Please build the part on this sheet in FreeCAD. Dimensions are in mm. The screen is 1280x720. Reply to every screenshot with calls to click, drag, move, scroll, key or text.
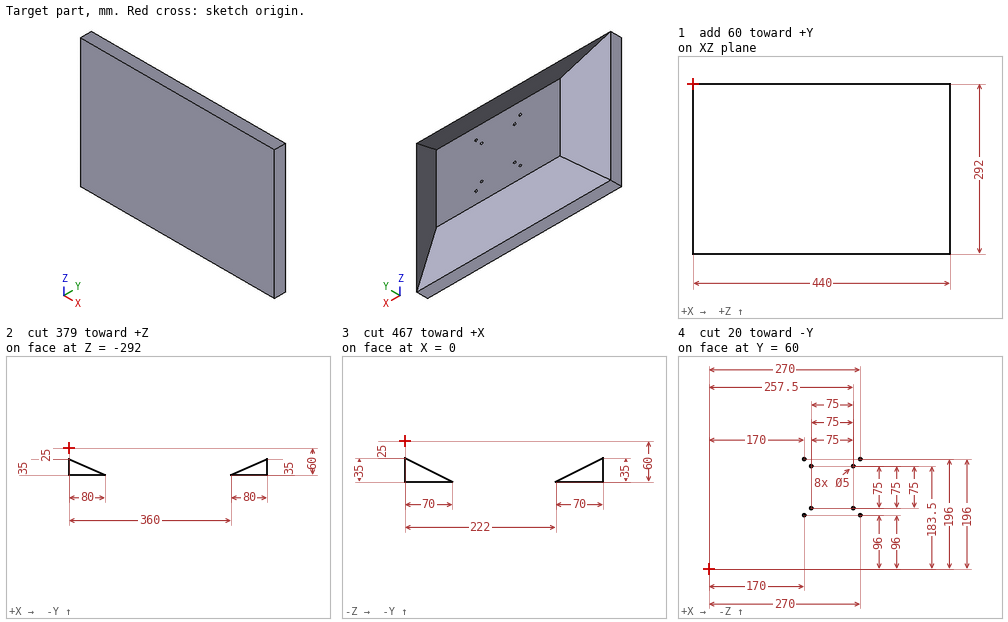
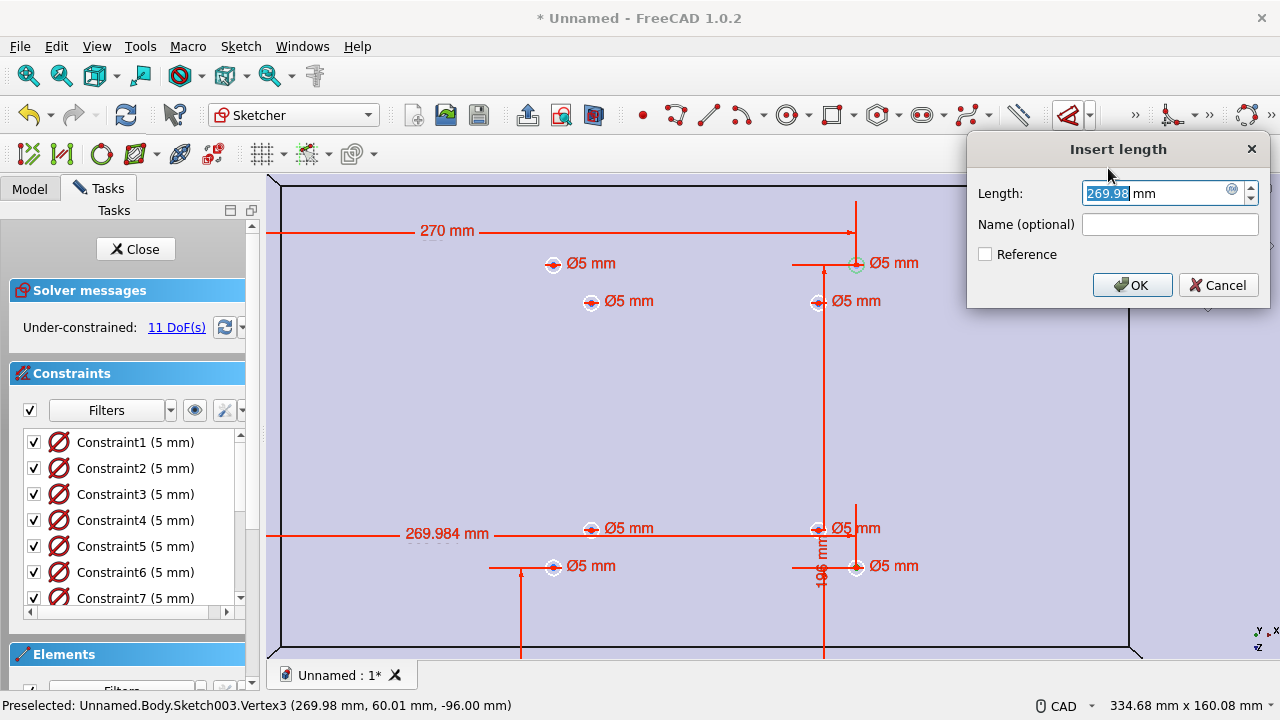
text(270)
key(Return)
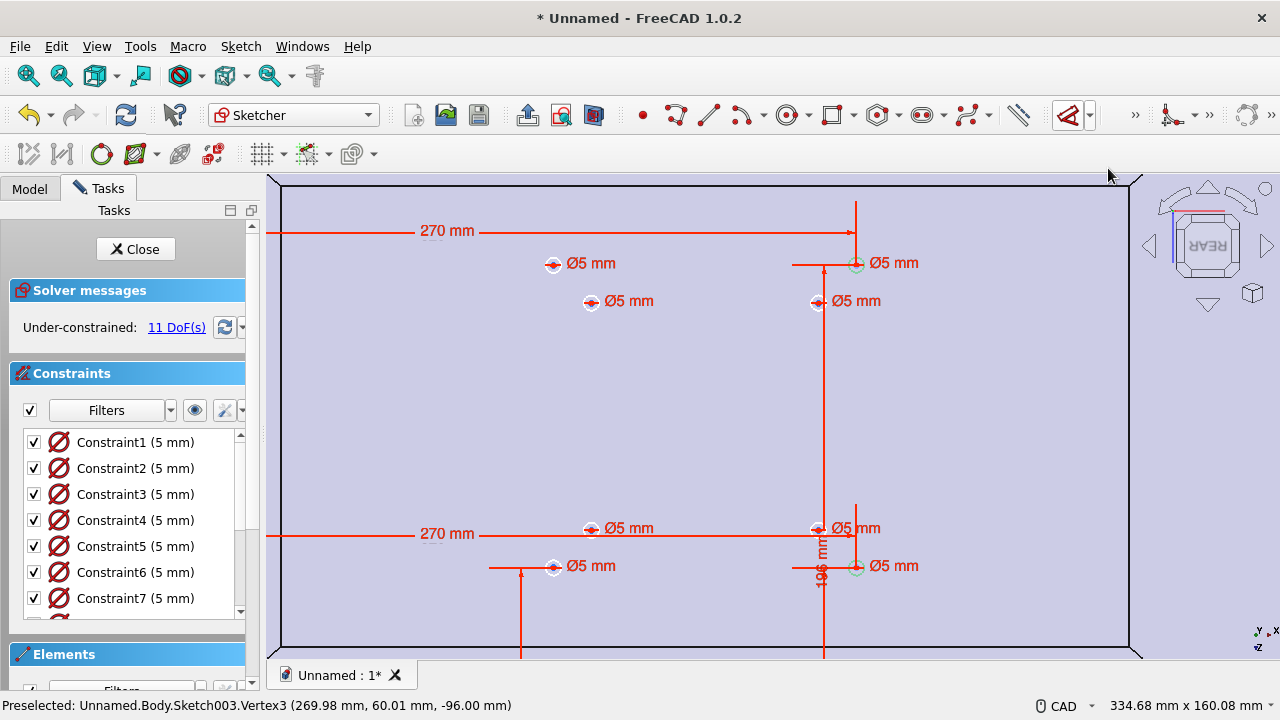
click(553, 568)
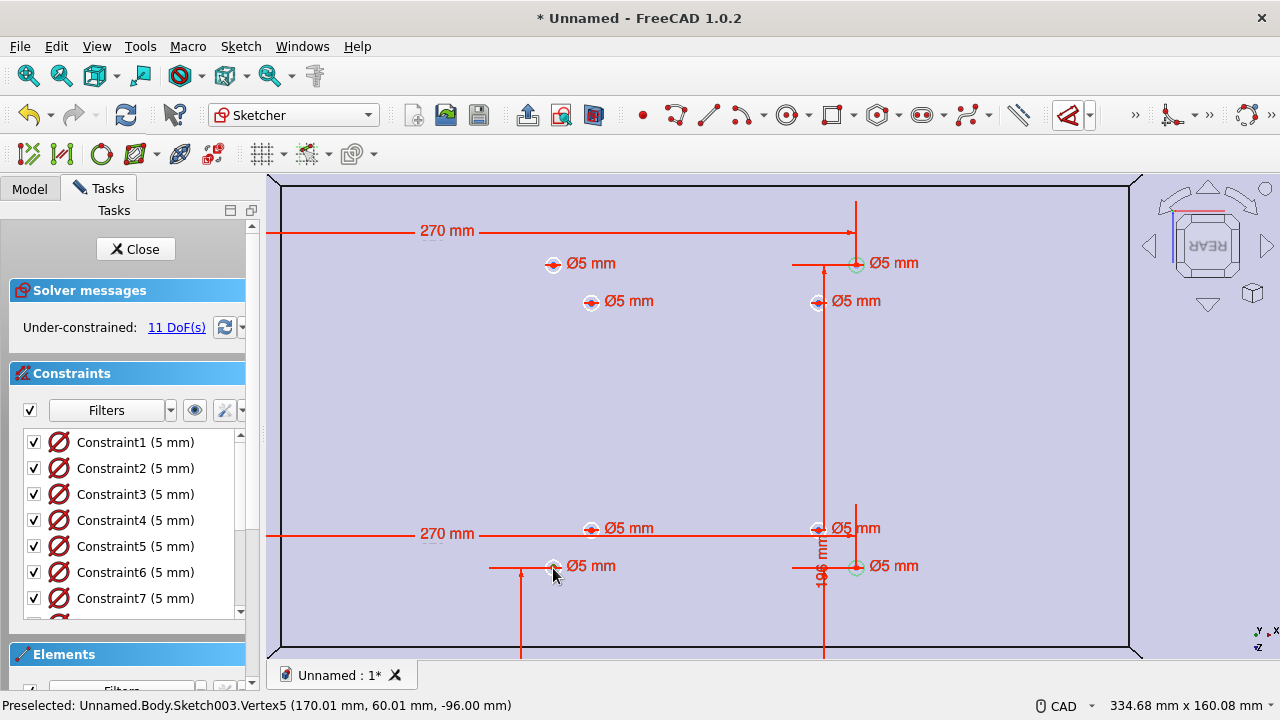
key(l)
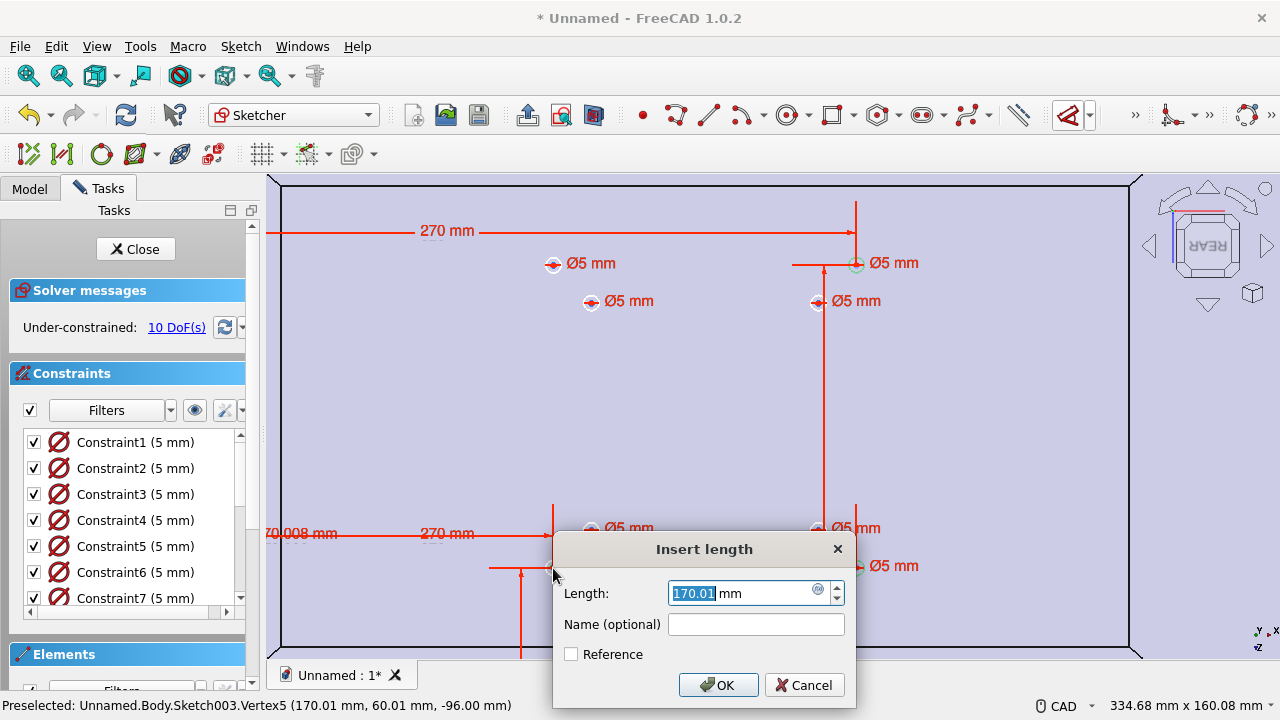
text(170)
key(Return)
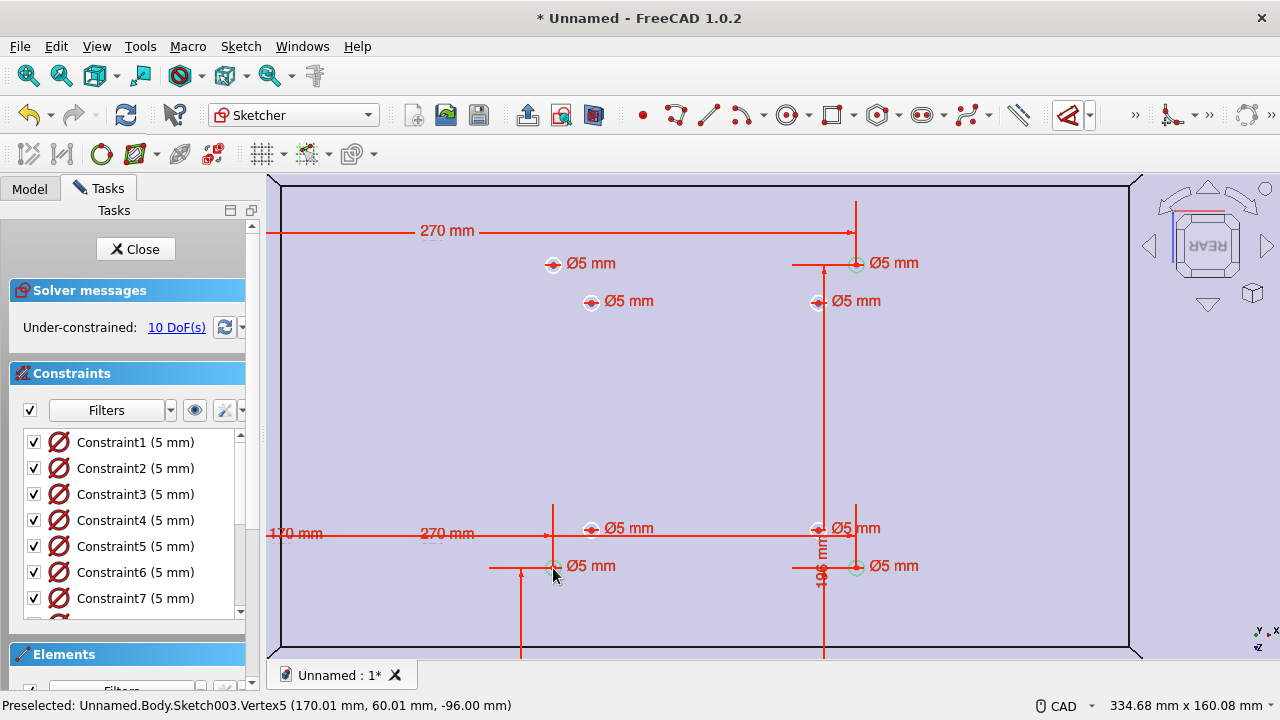
click(553, 265)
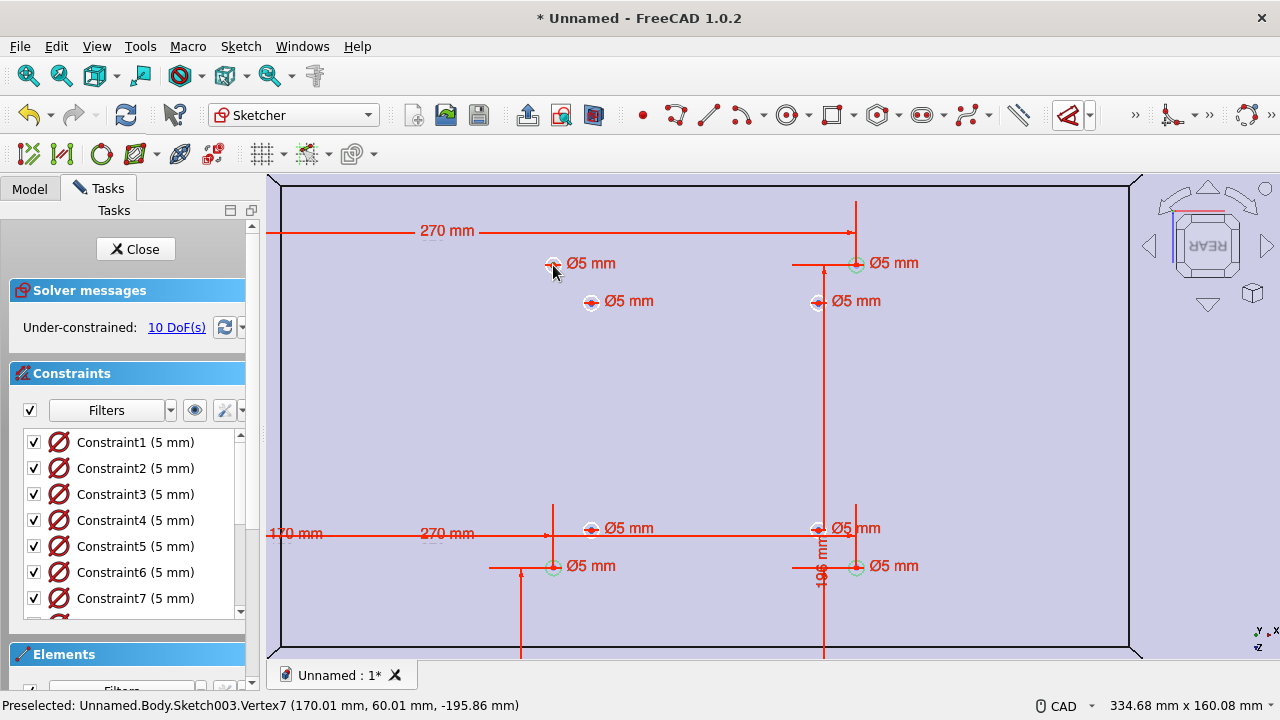
key(l)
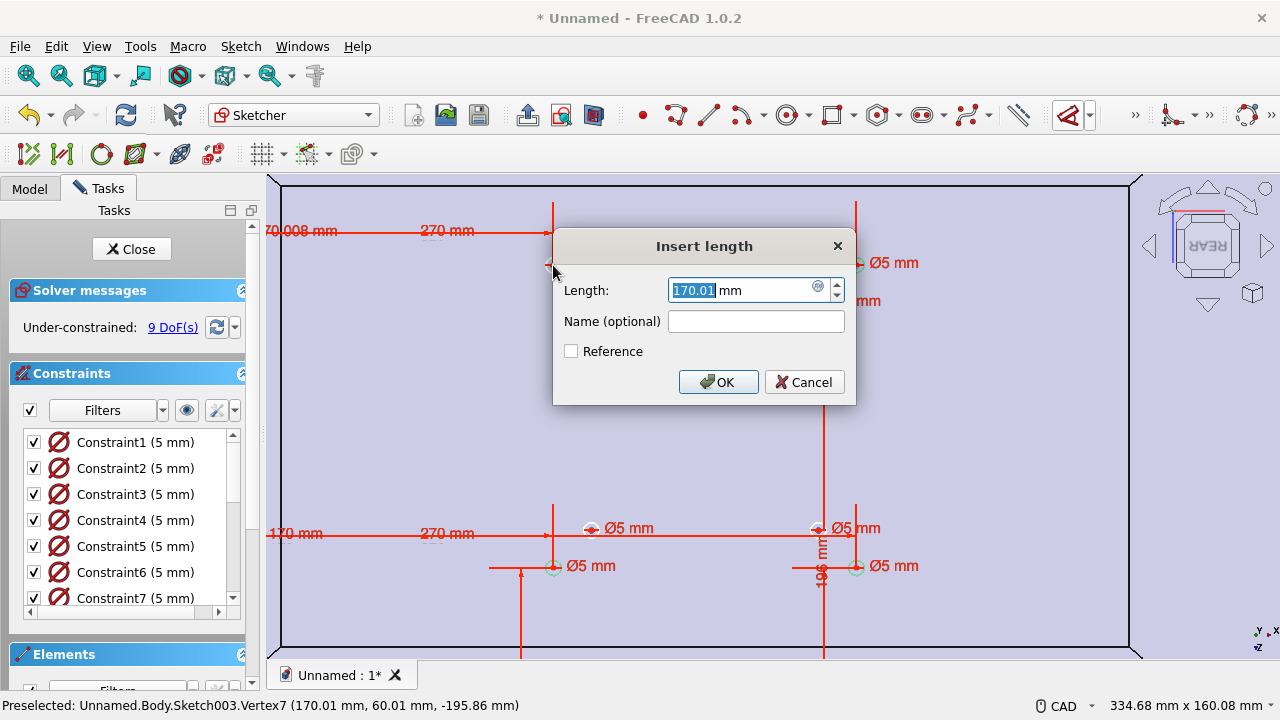
text(170)
key(Return)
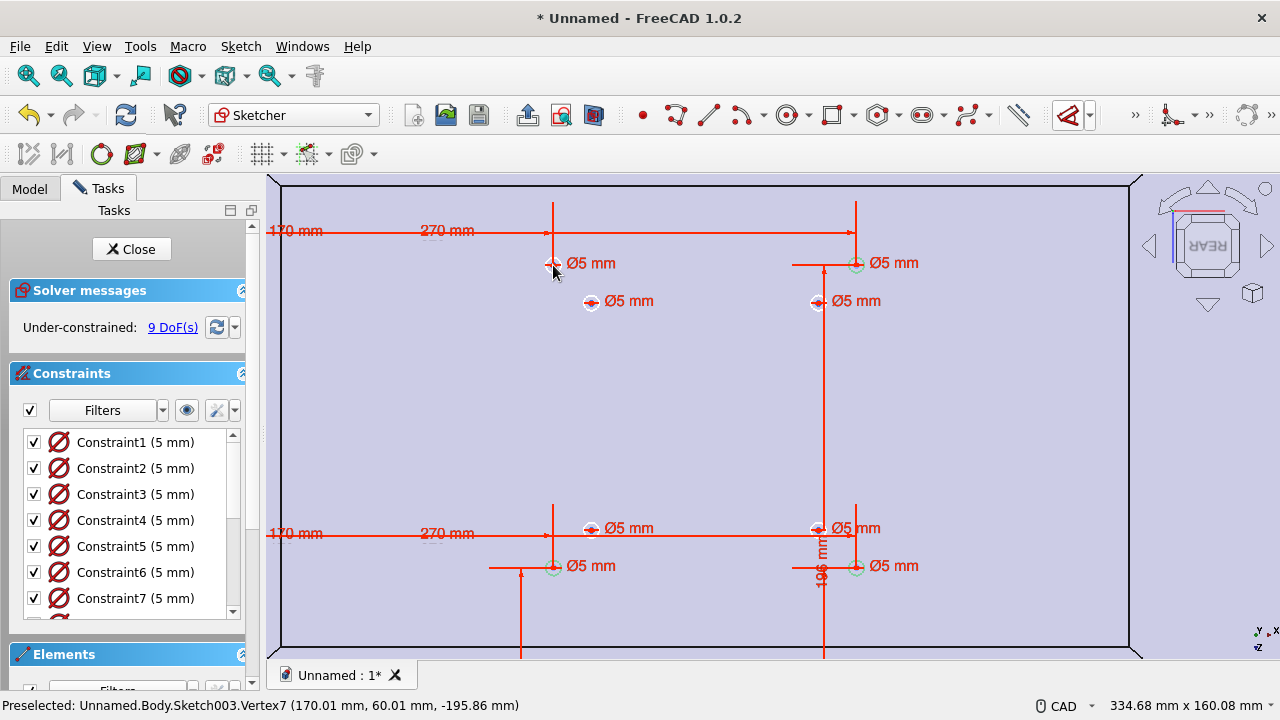
click(553, 265)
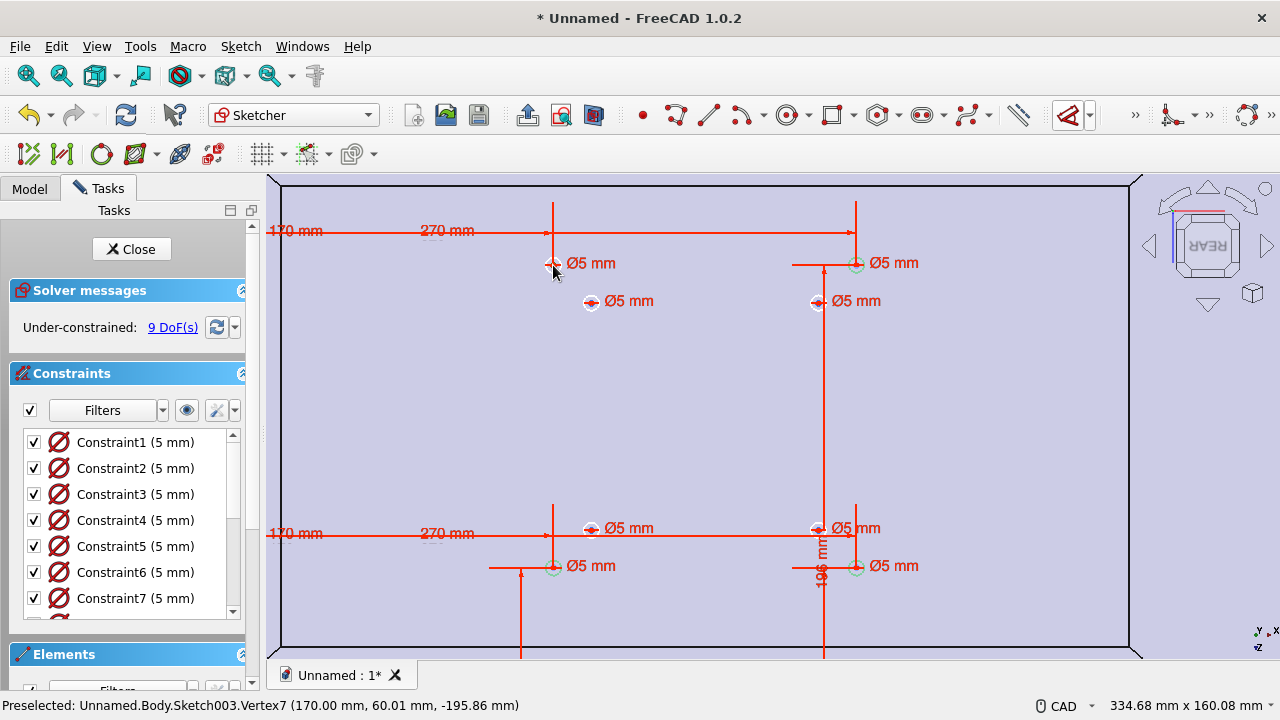
click(1090, 116)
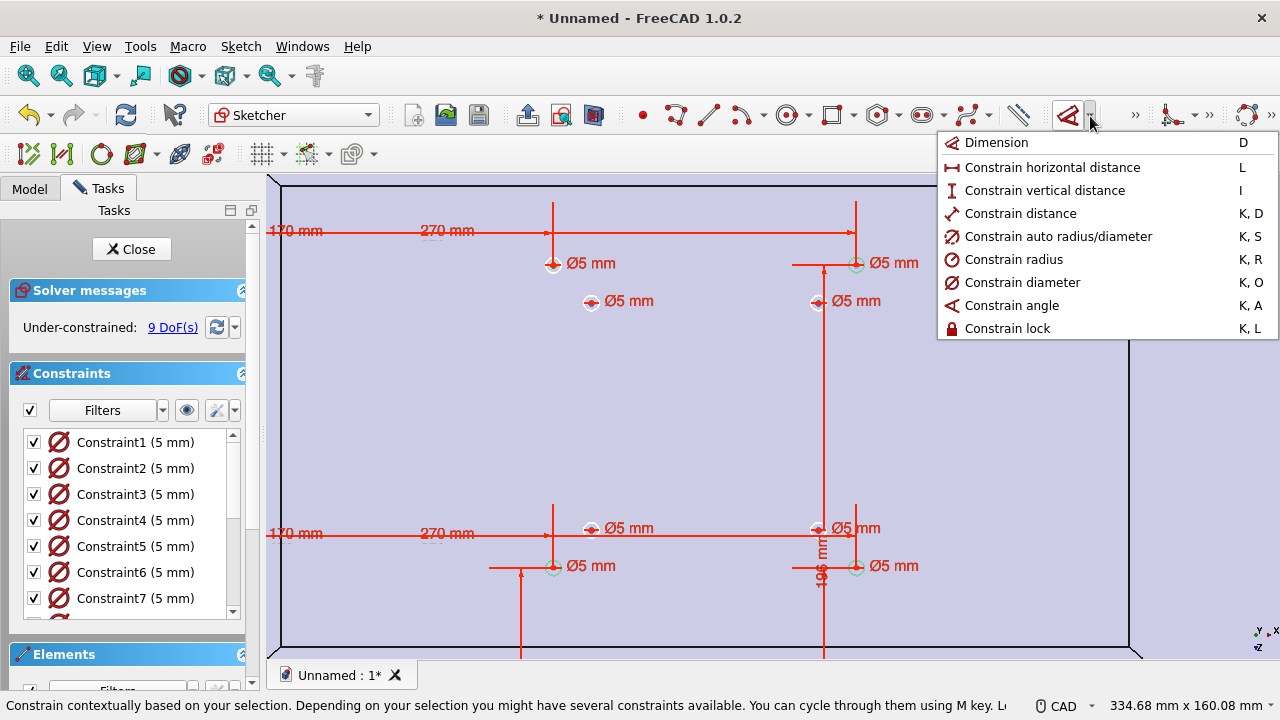
click(1108, 190)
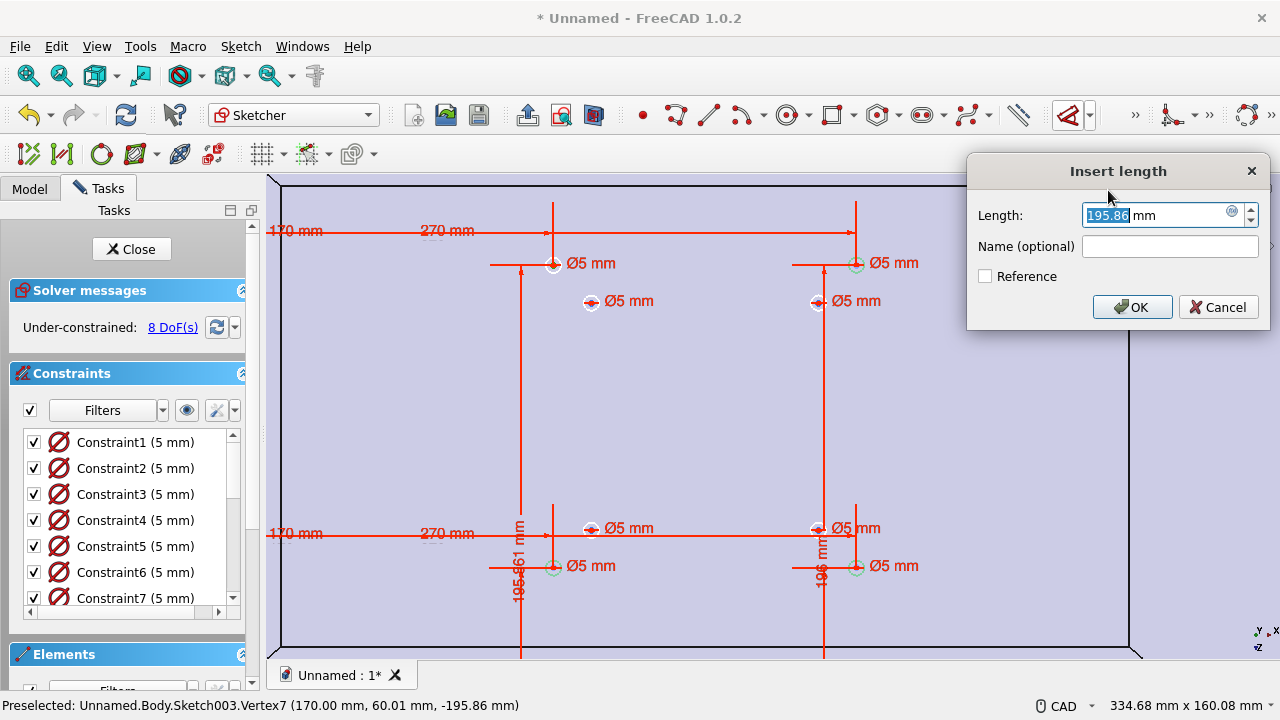
text(196)
key(Return)